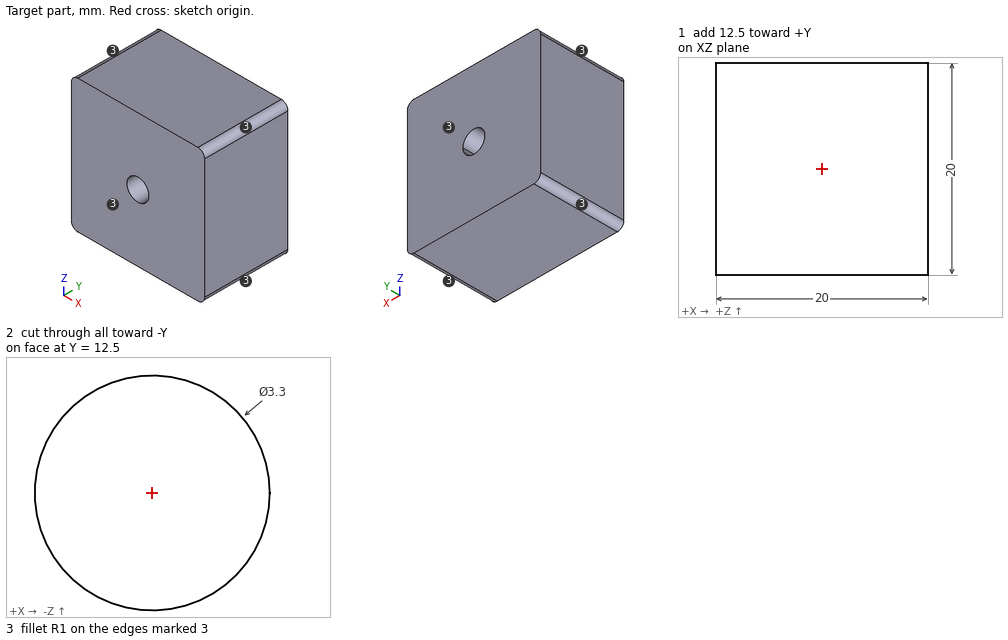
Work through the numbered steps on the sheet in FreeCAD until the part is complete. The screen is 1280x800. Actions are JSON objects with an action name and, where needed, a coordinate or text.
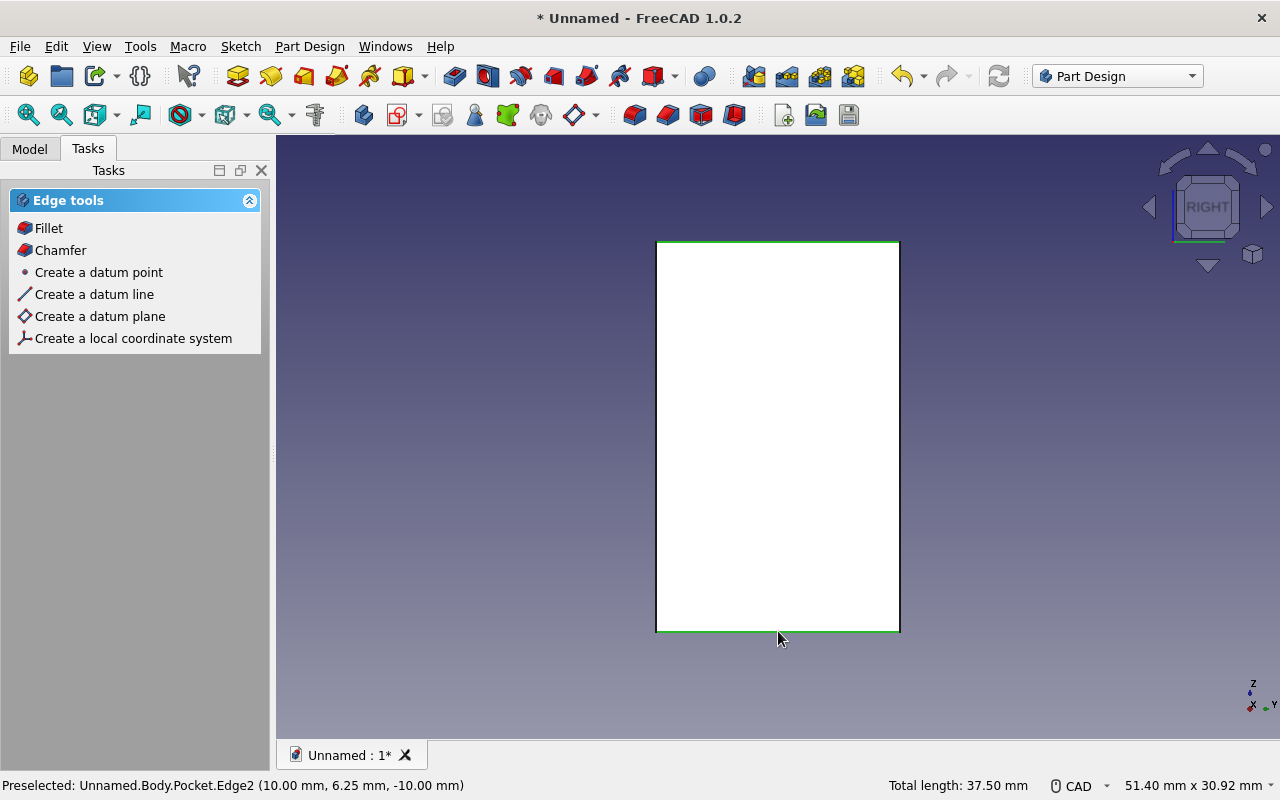
{"action": "key", "text": "5"}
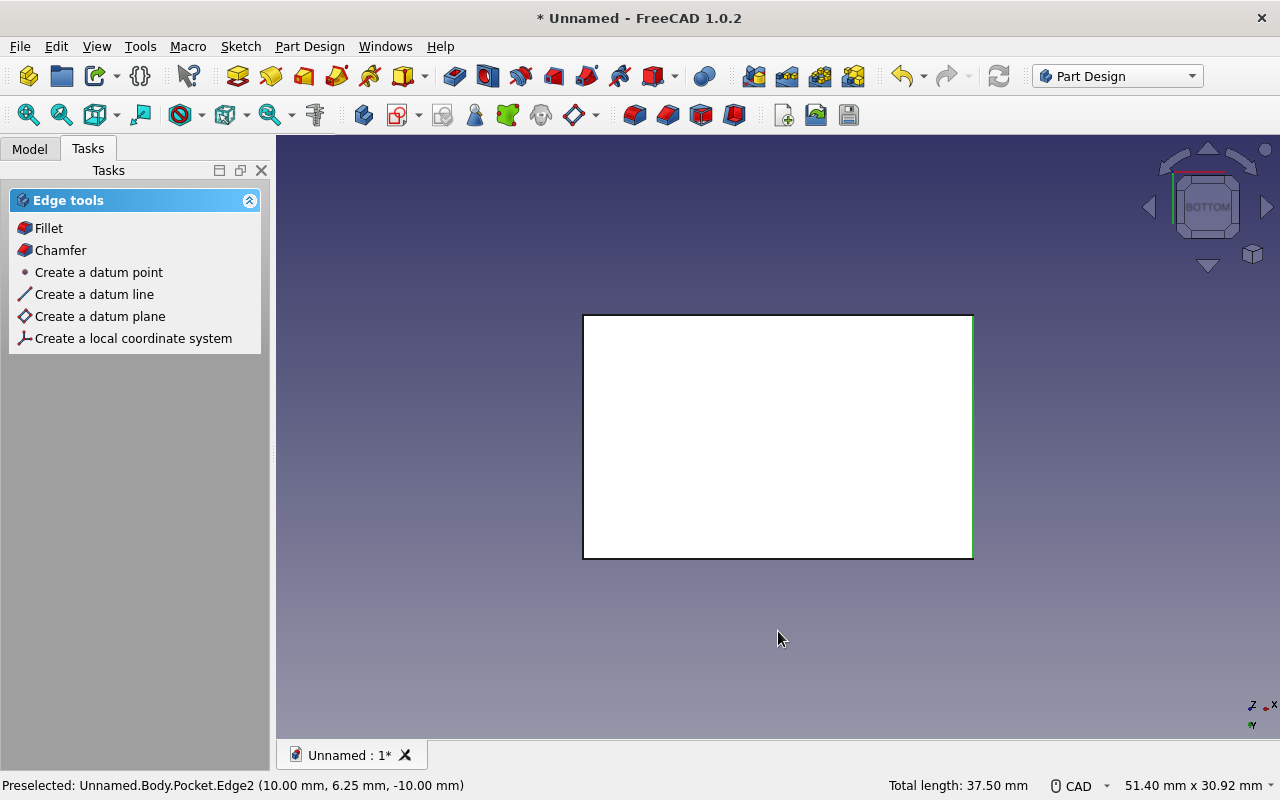
{"action": "left_click", "coordinate": [29, 116]}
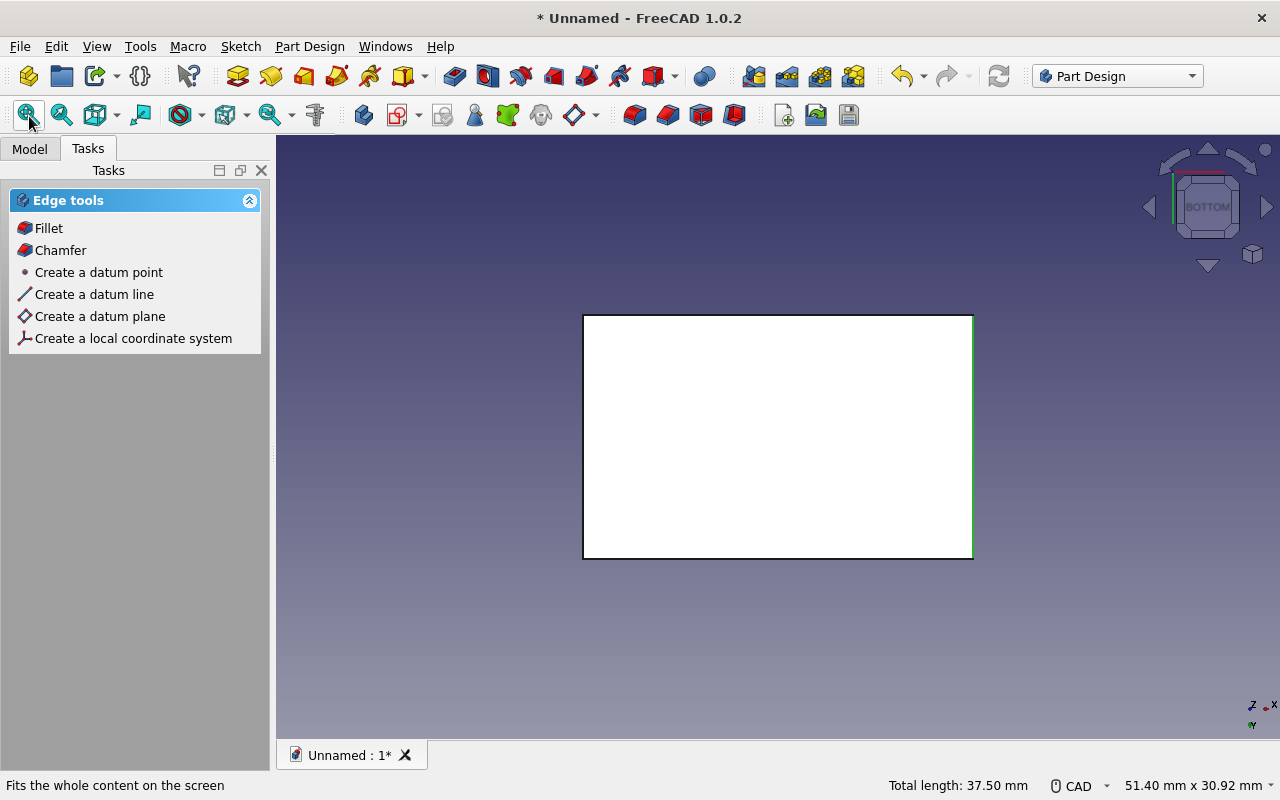
{"action": "left_click", "coordinate": [583, 436], "text": "ctrl"}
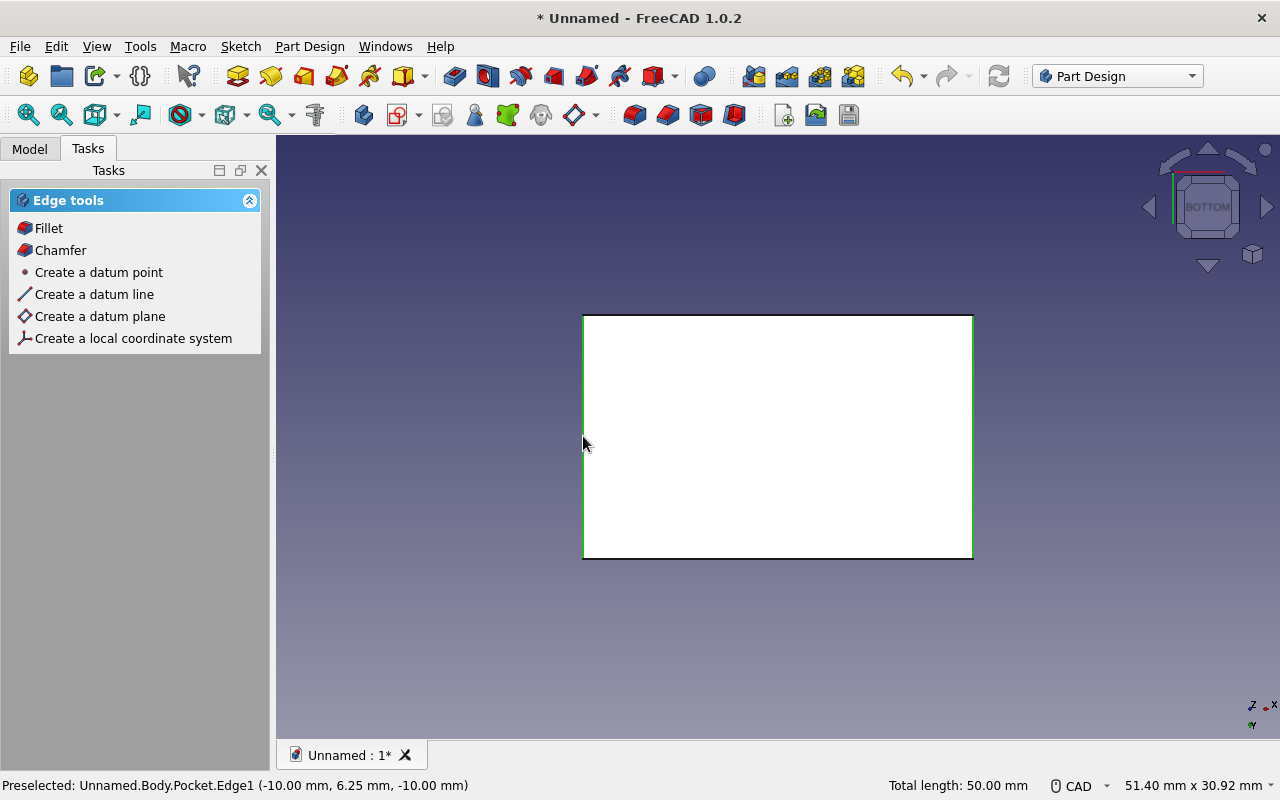
{"action": "left_click", "coordinate": [635, 116]}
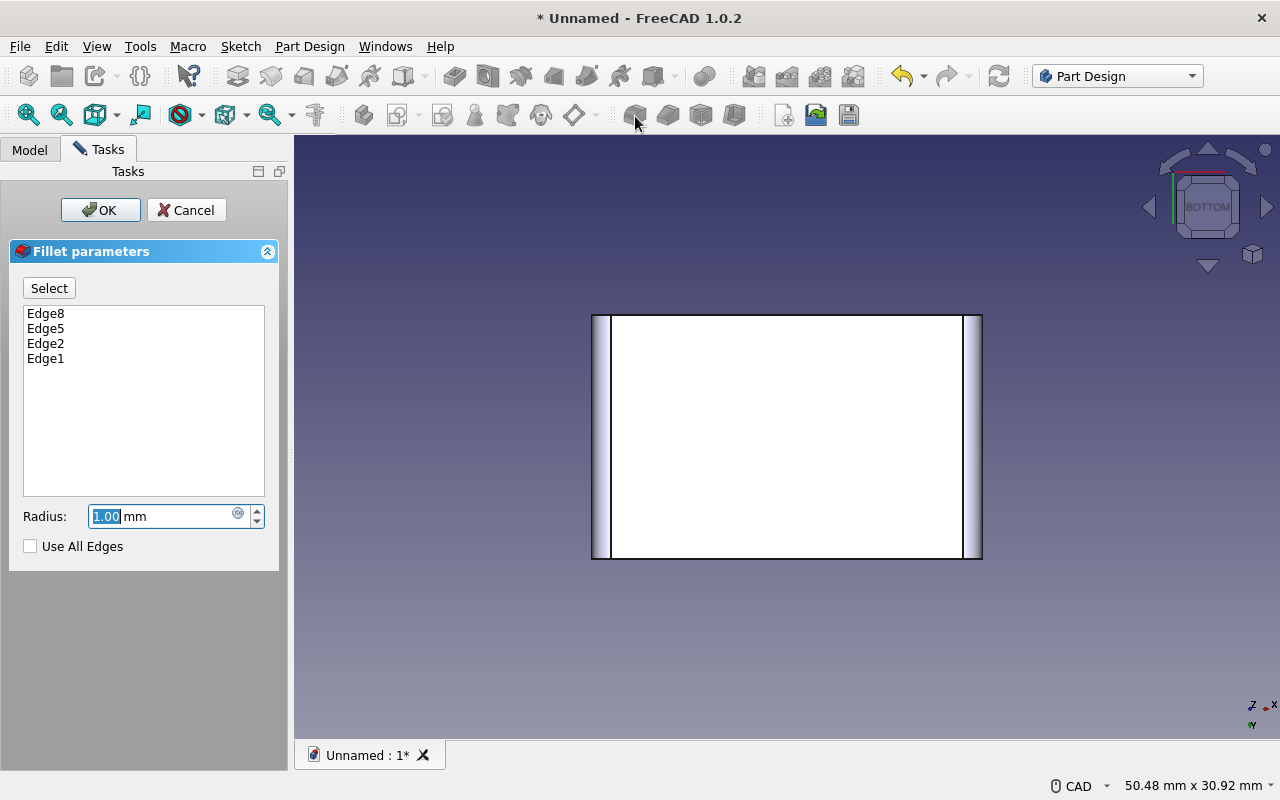
{"action": "type", "text": "1"}
{"action": "key", "text": "Tab"}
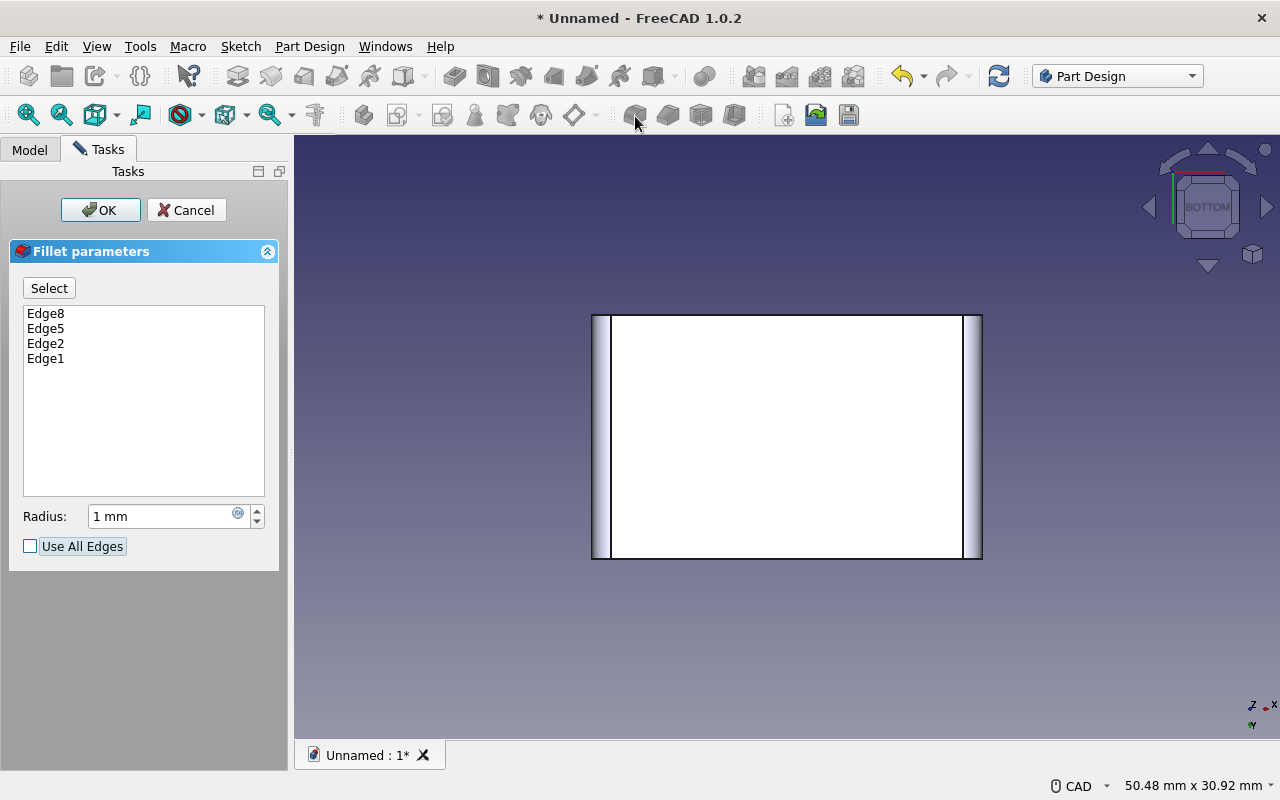
{"action": "left_click", "coordinate": [101, 210]}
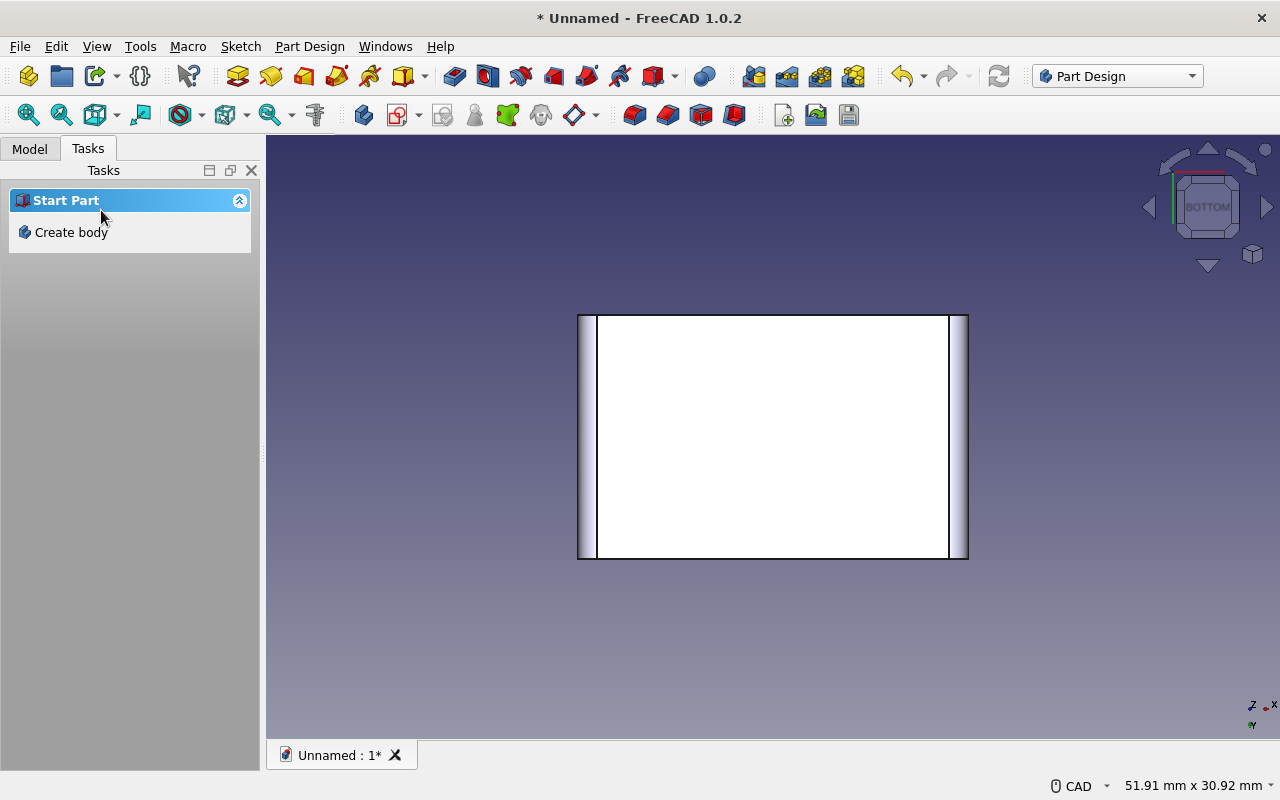
{"action": "key", "text": "0"}